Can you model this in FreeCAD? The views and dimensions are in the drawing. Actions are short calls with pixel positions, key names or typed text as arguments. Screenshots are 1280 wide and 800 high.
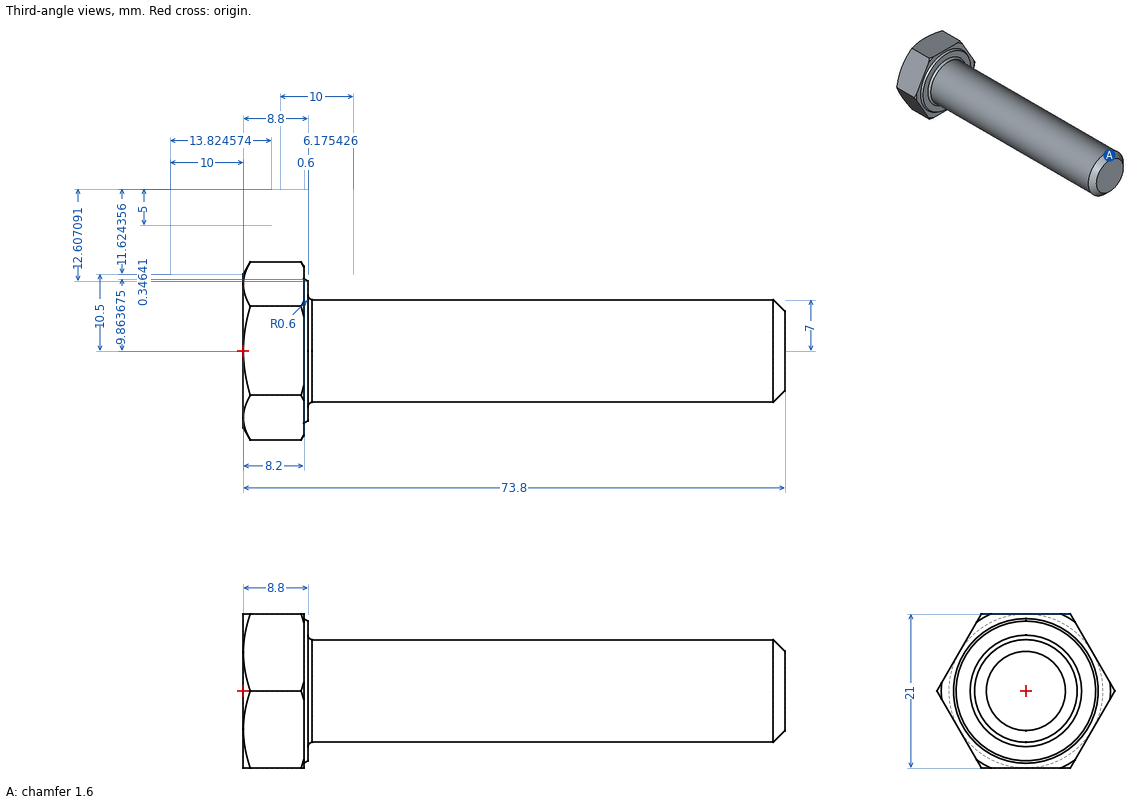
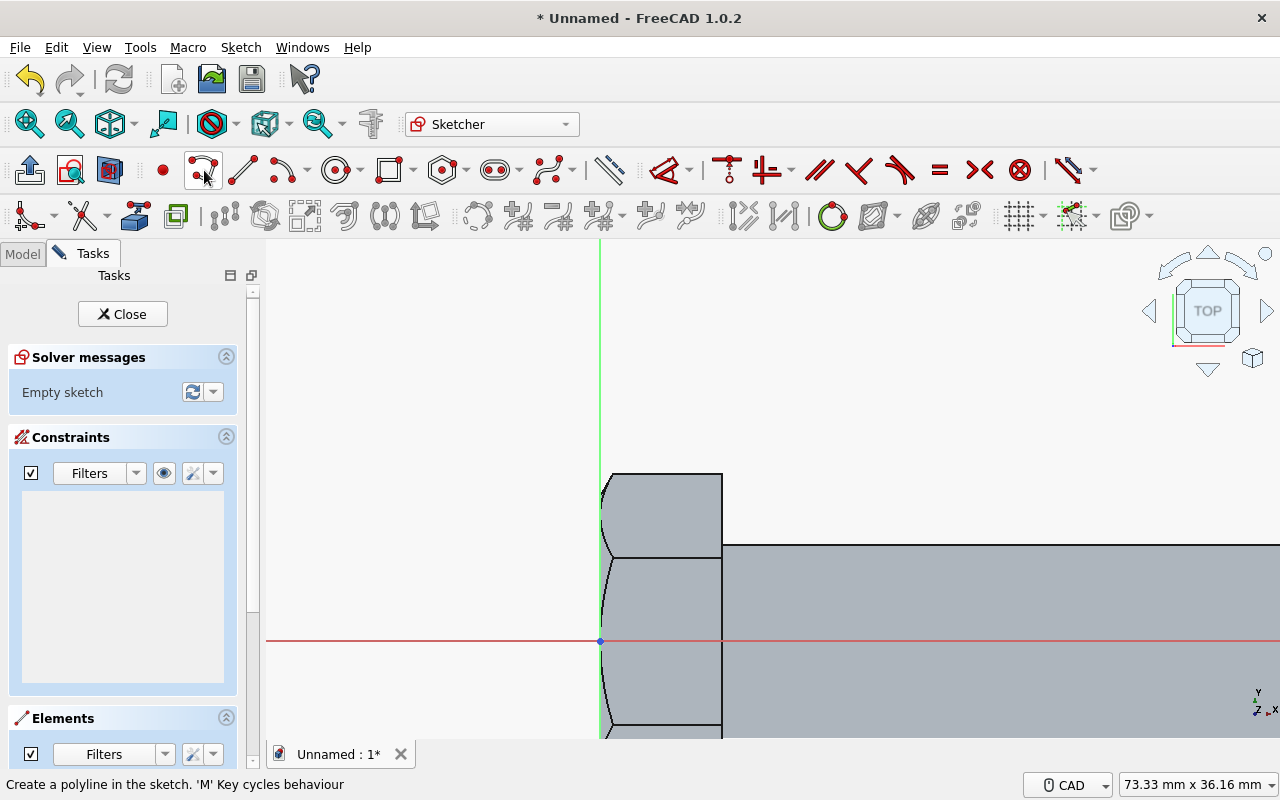
click(722, 496)
click(807, 496)
click(807, 335)
click(669, 335)
click(669, 405)
click(722, 497)
key(Escape)
key(Escape)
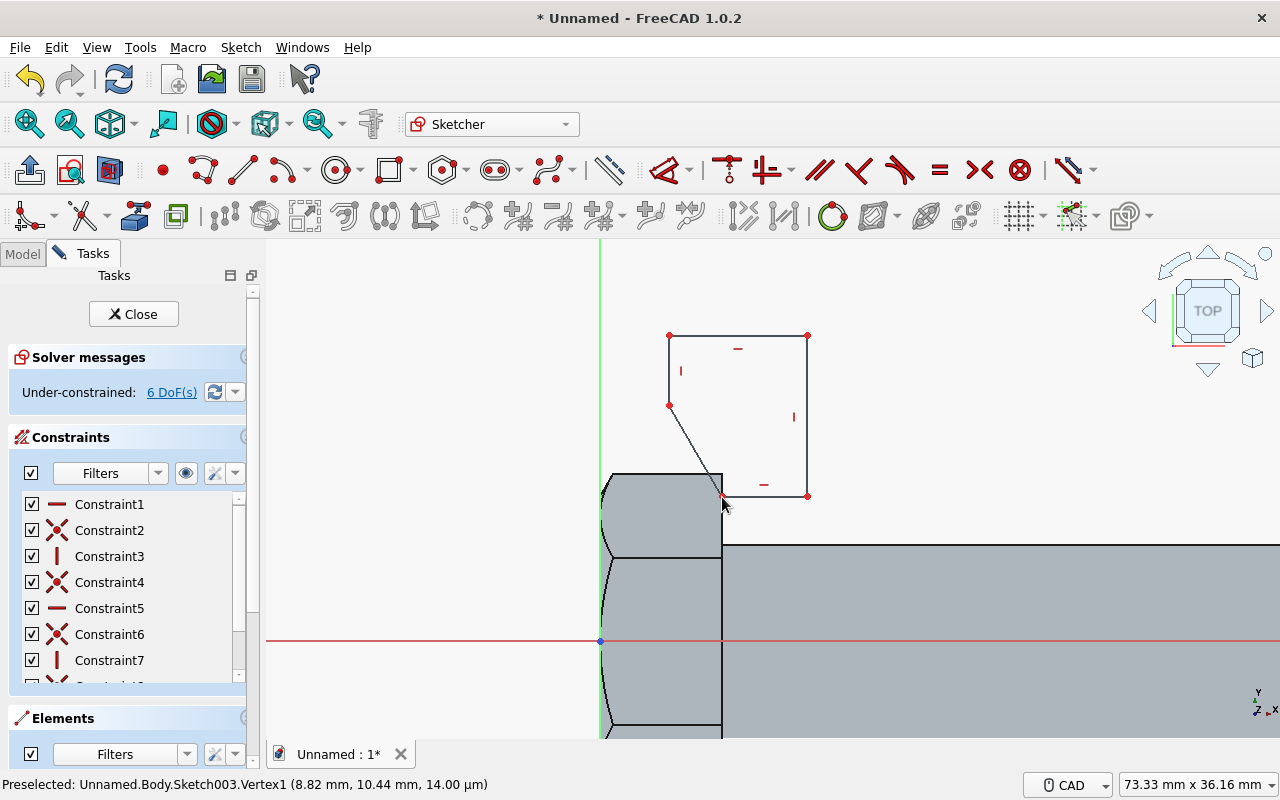
click(664, 170)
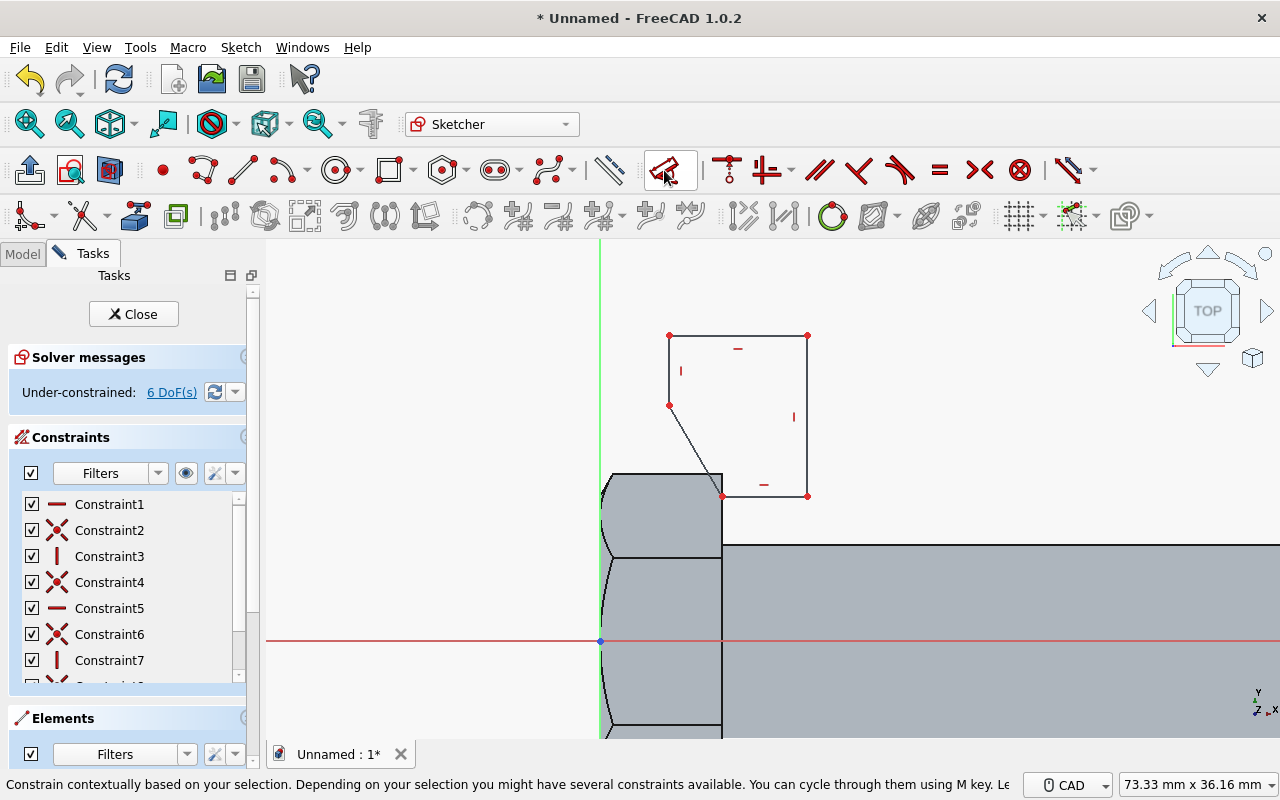
click(669, 357)
click(635, 371)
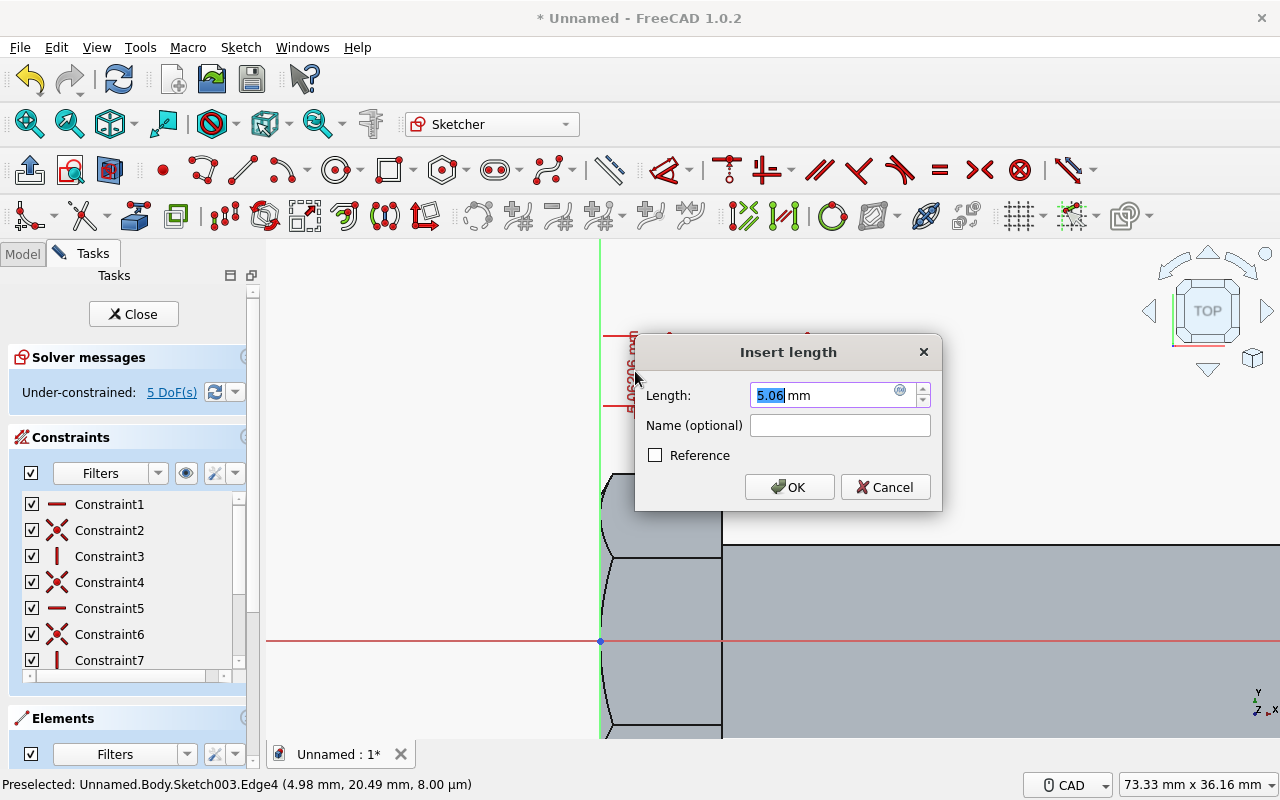
text(5)
key(Return)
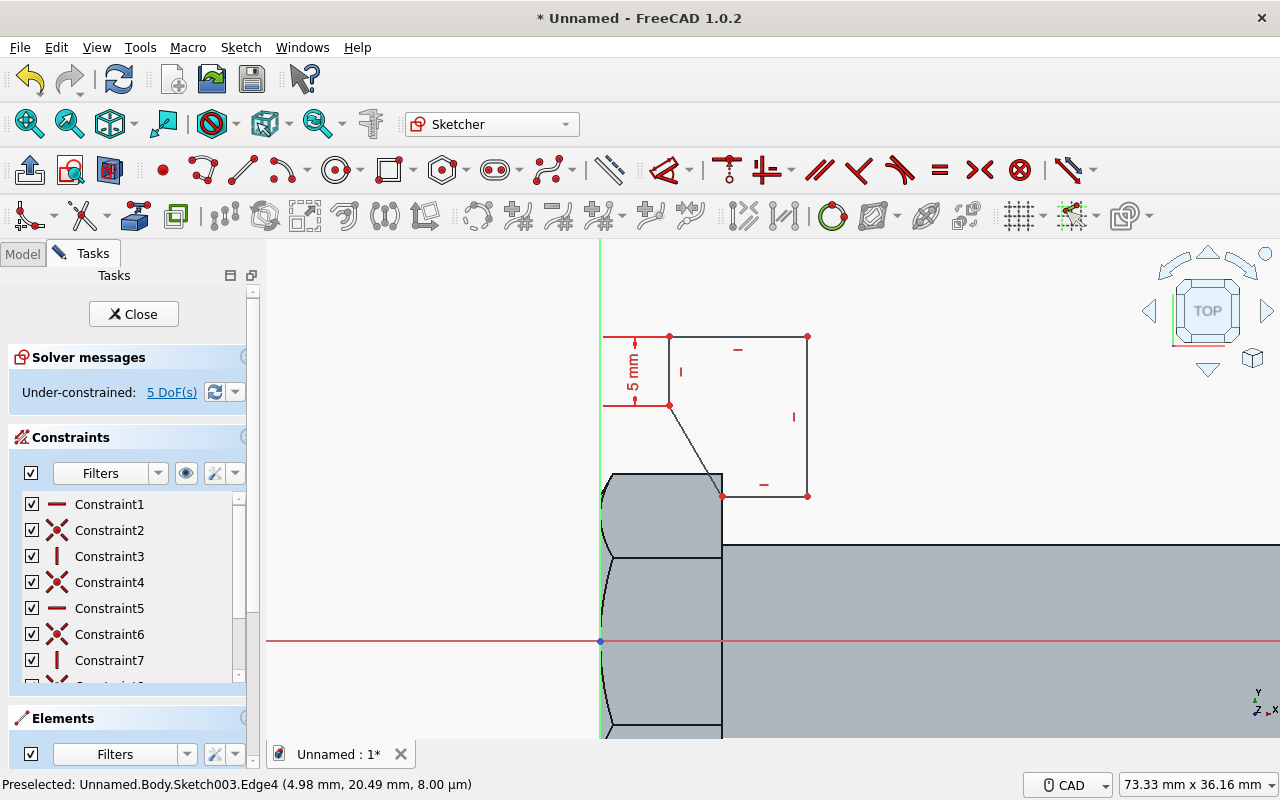
click(766, 337)
click(738, 303)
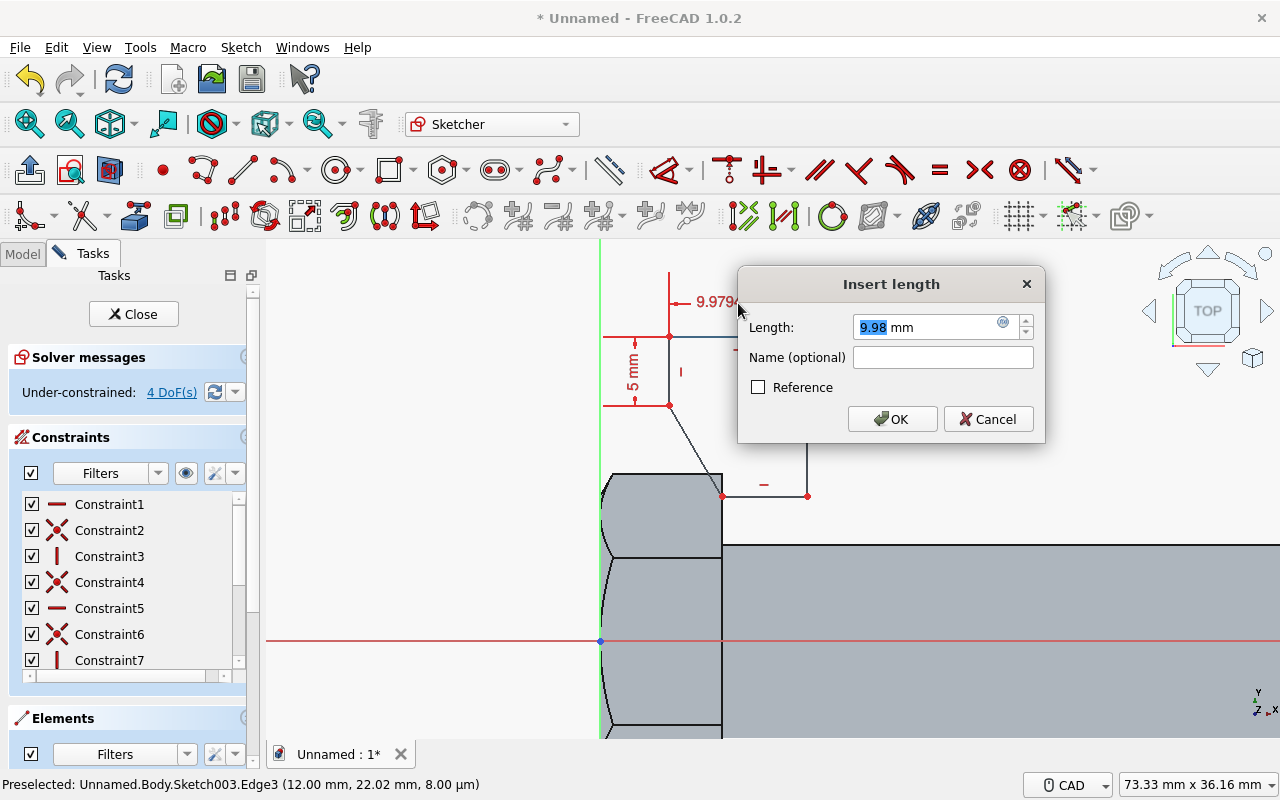
text(10)
key(Return)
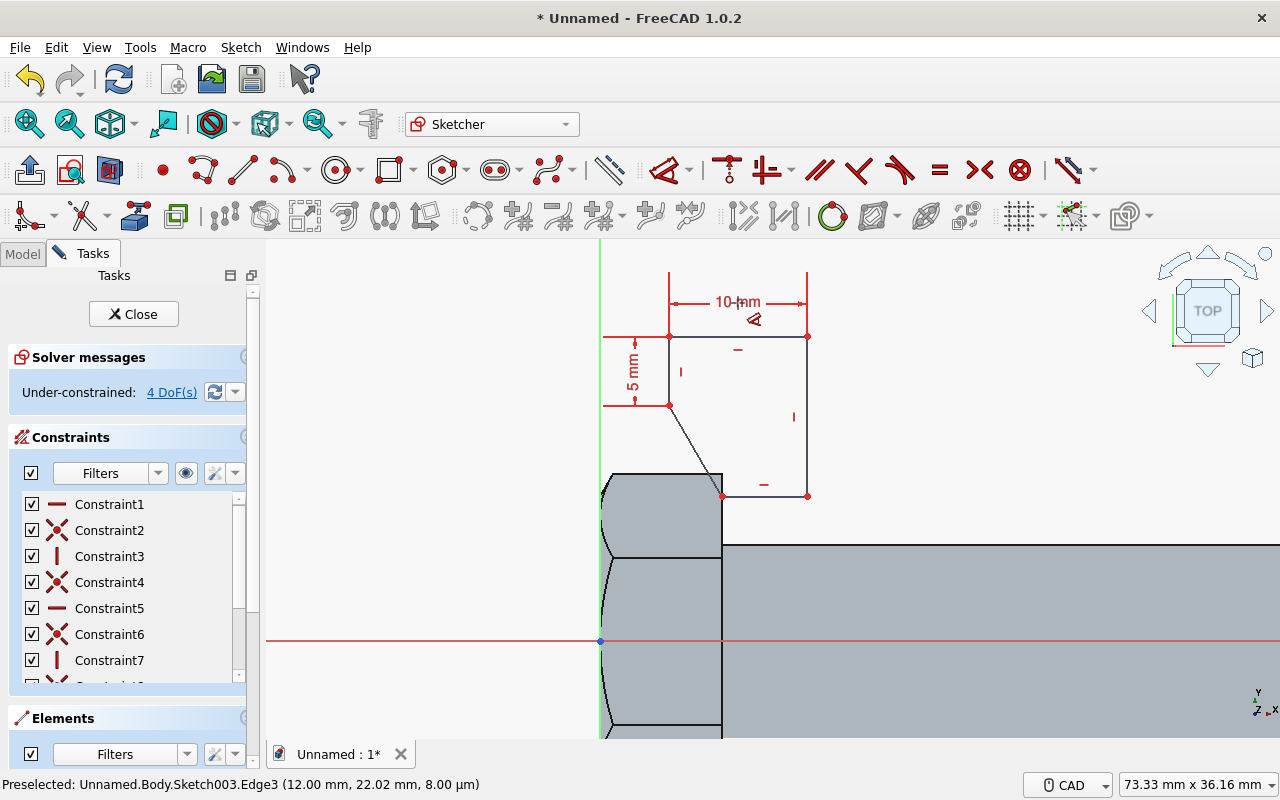
click(722, 497)
click(661, 675)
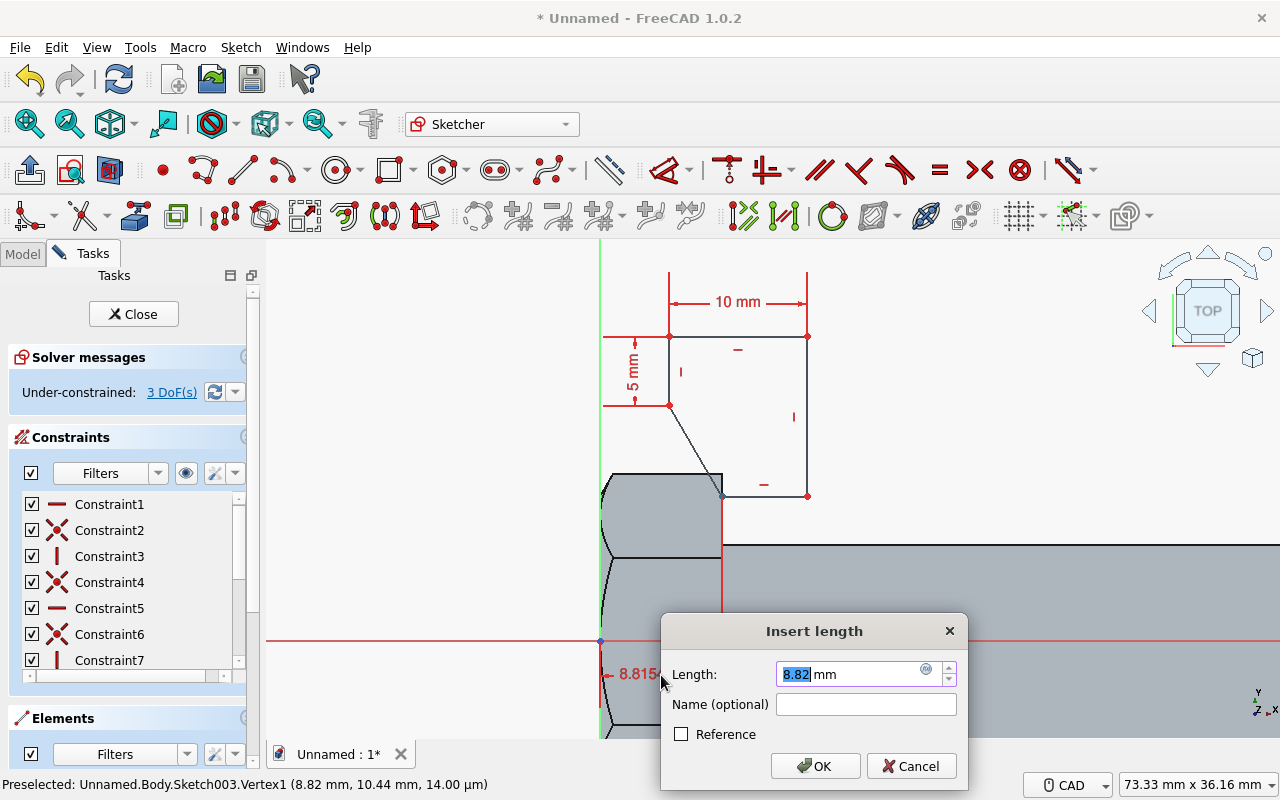
text(8.8)
key(Return)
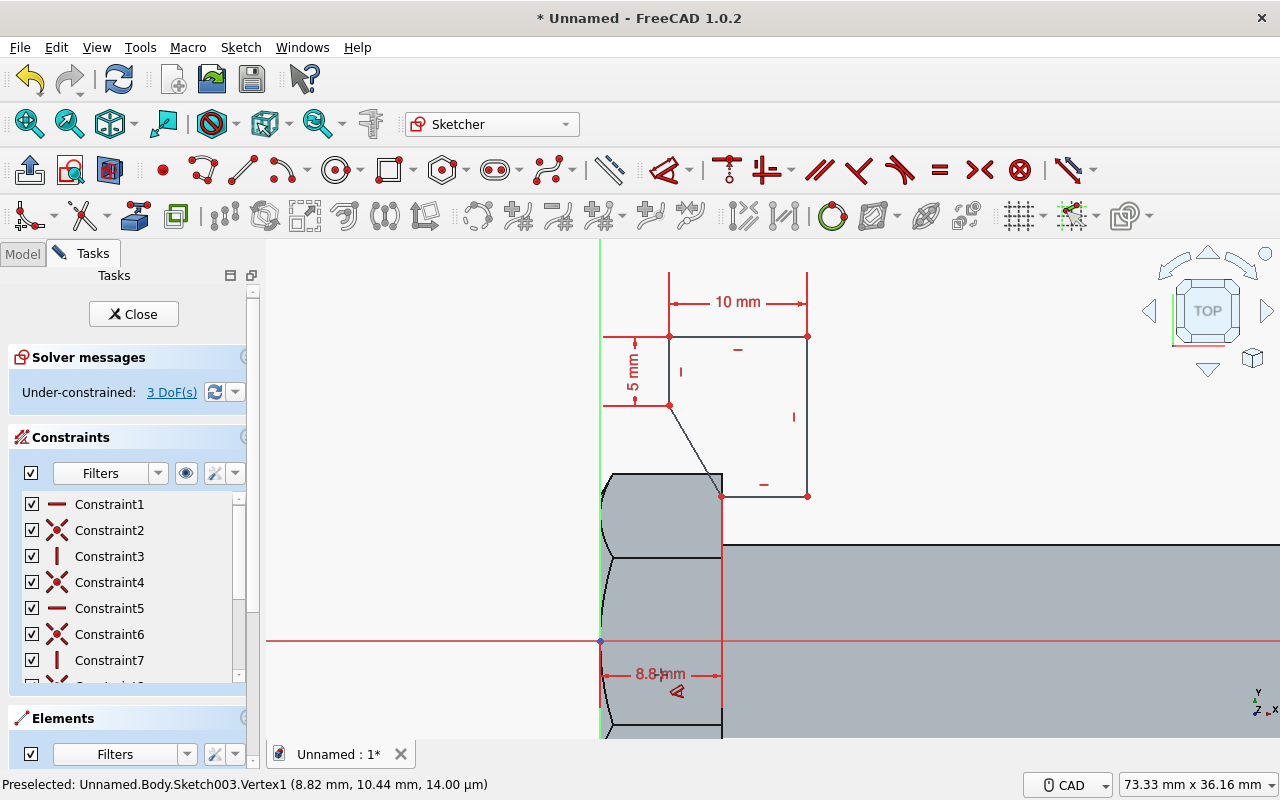
click(722, 497)
click(566, 569)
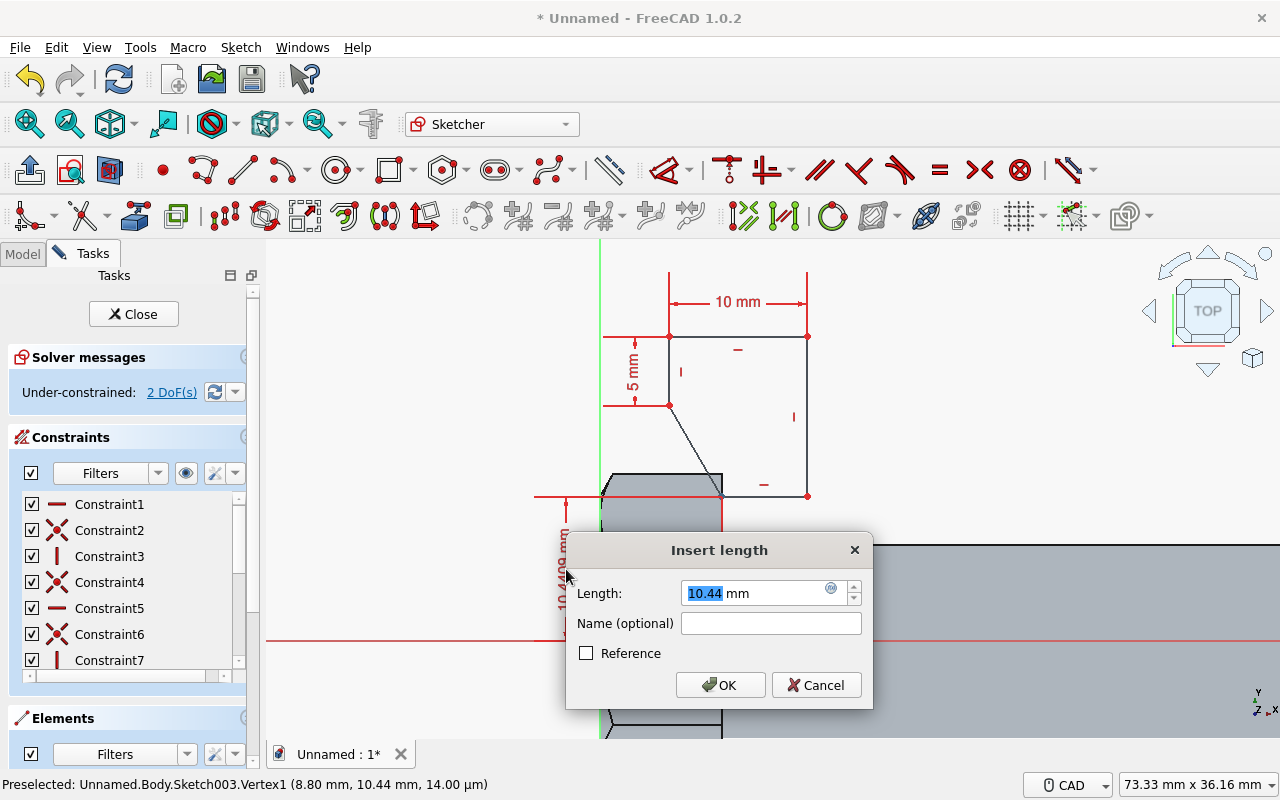
text(10.5)
key(Return)